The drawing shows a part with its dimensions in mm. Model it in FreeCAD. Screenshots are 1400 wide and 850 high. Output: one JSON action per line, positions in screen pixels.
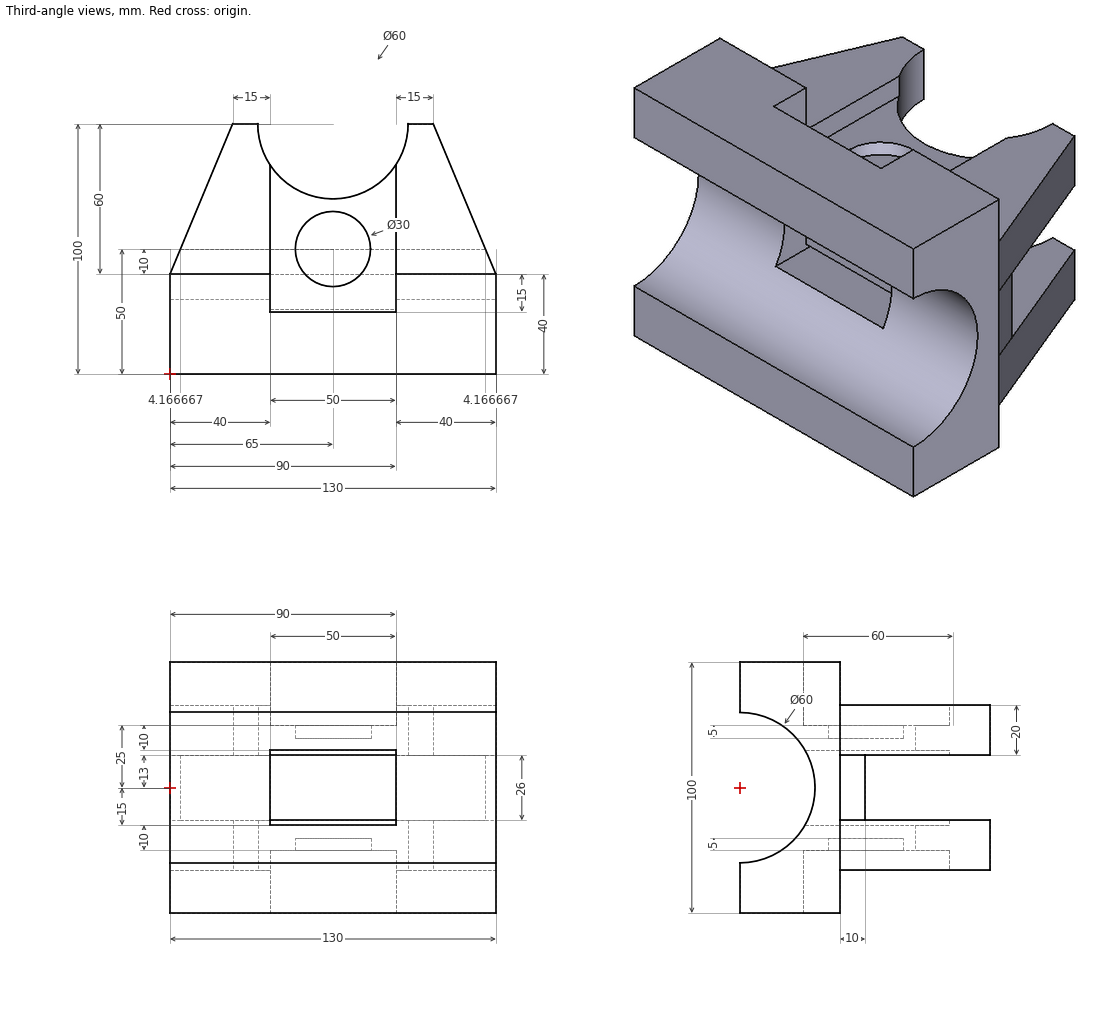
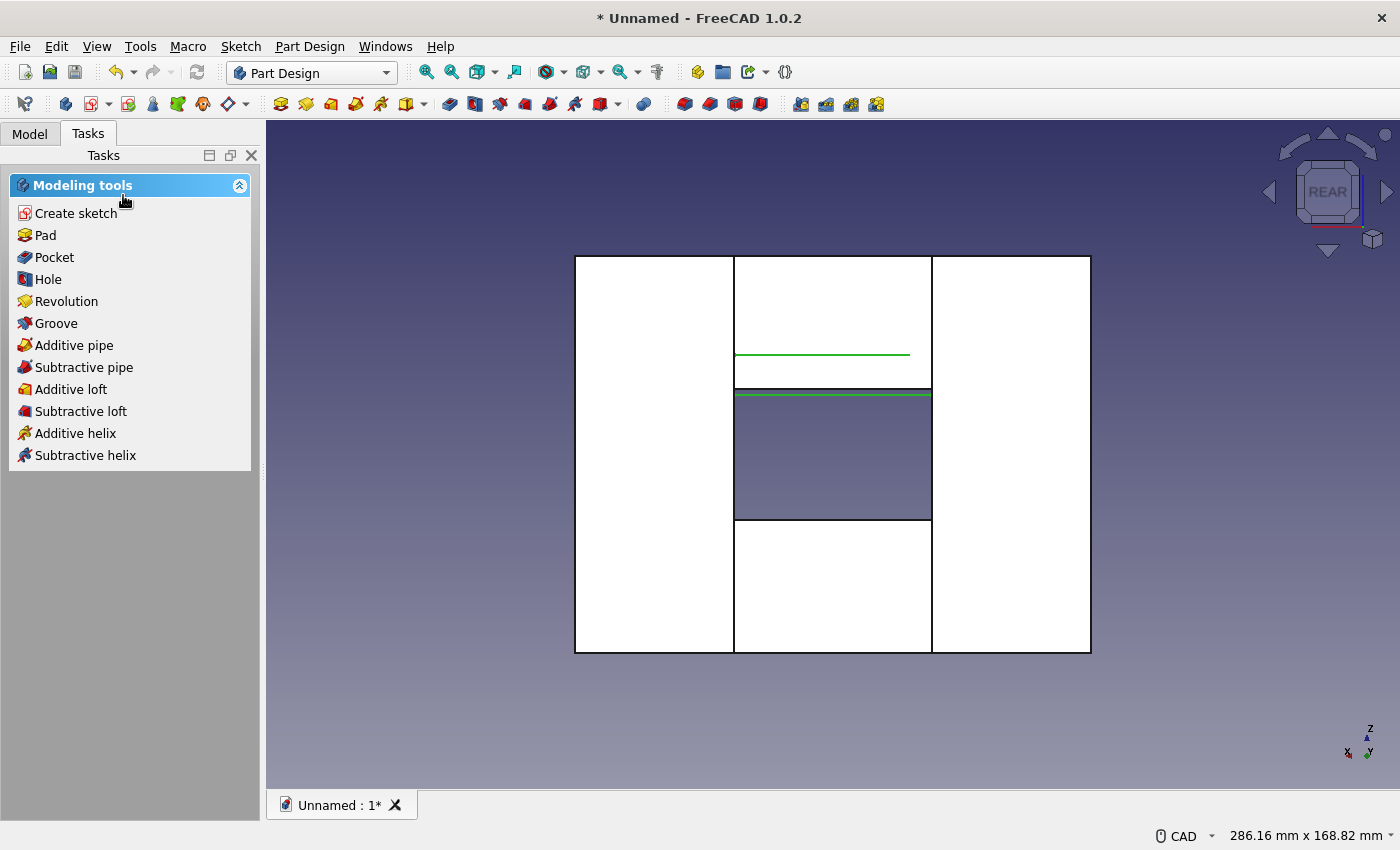
{"action": "left_click", "coordinate": [281, 104]}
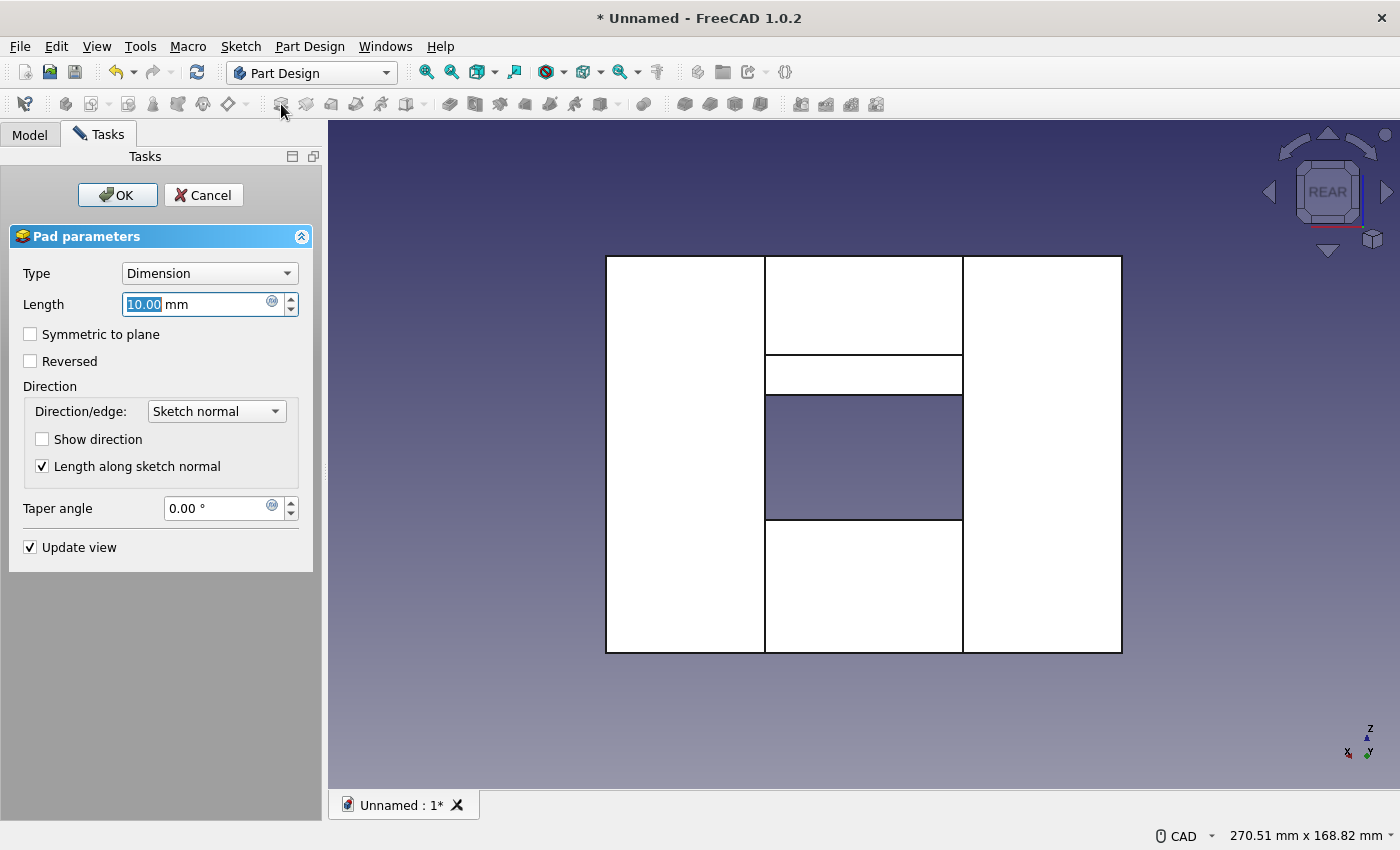
{"action": "type", "text": "60"}
{"action": "key", "text": "Tab"}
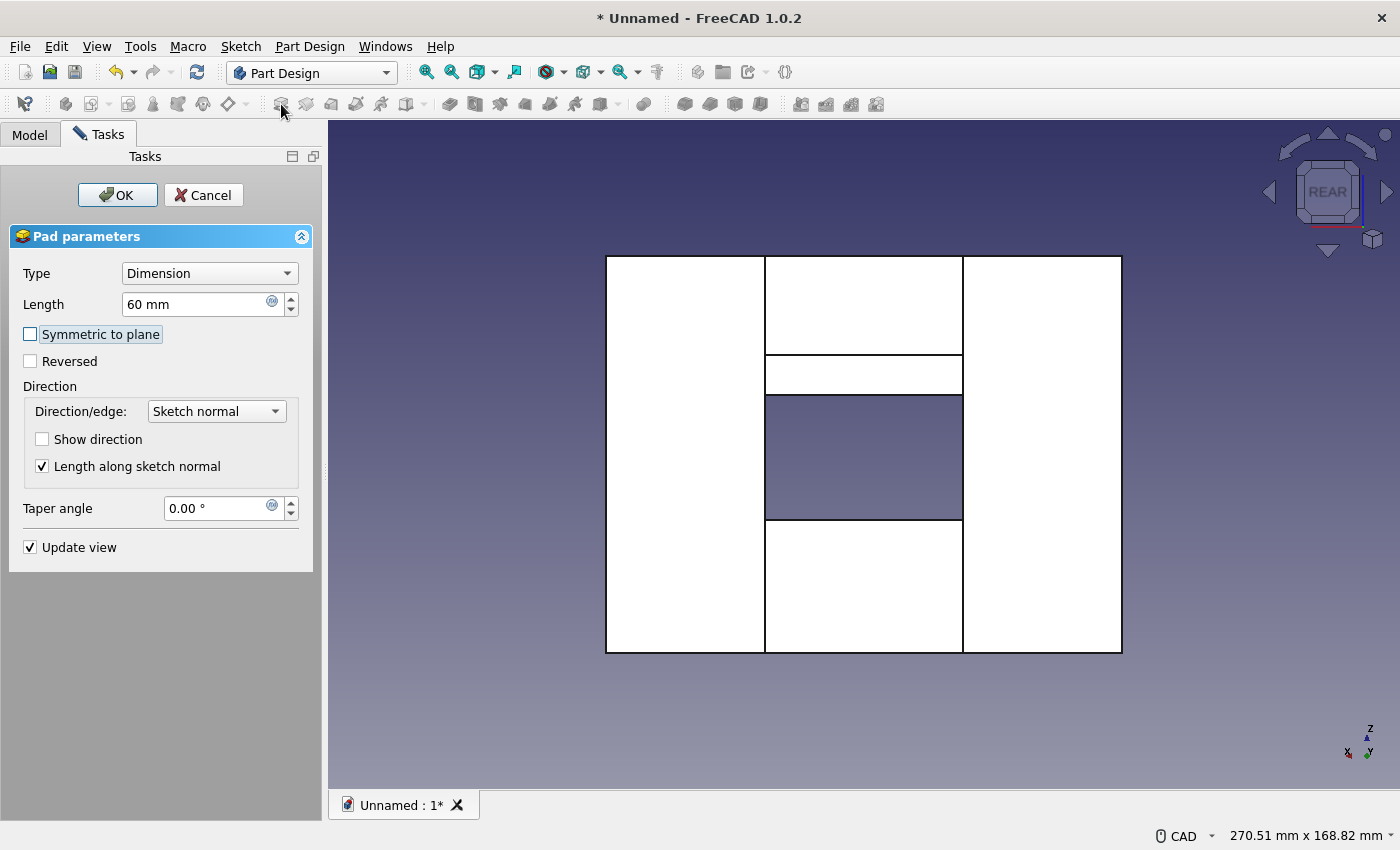
{"action": "left_click", "coordinate": [118, 195]}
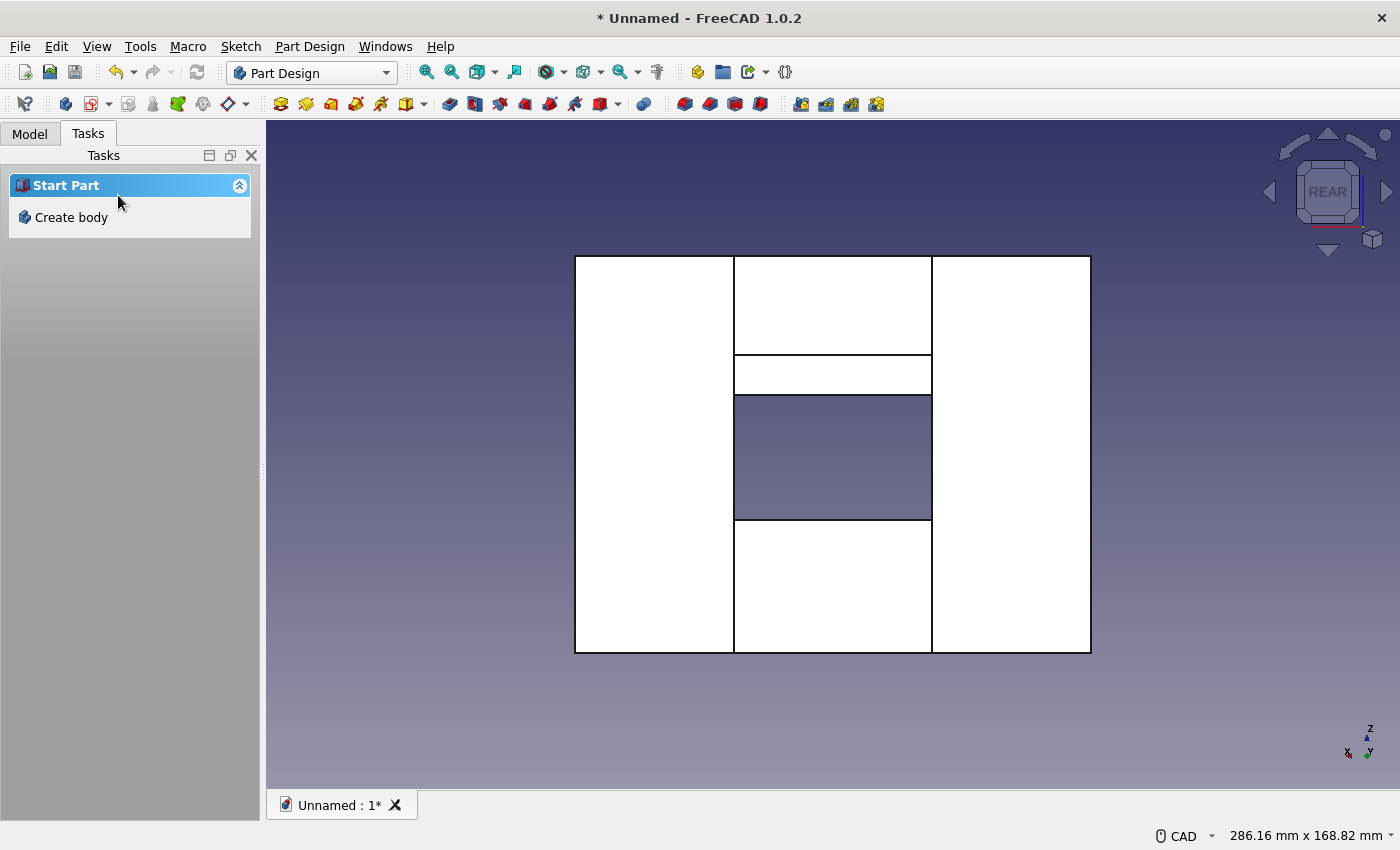
{"action": "left_click", "coordinate": [805, 585]}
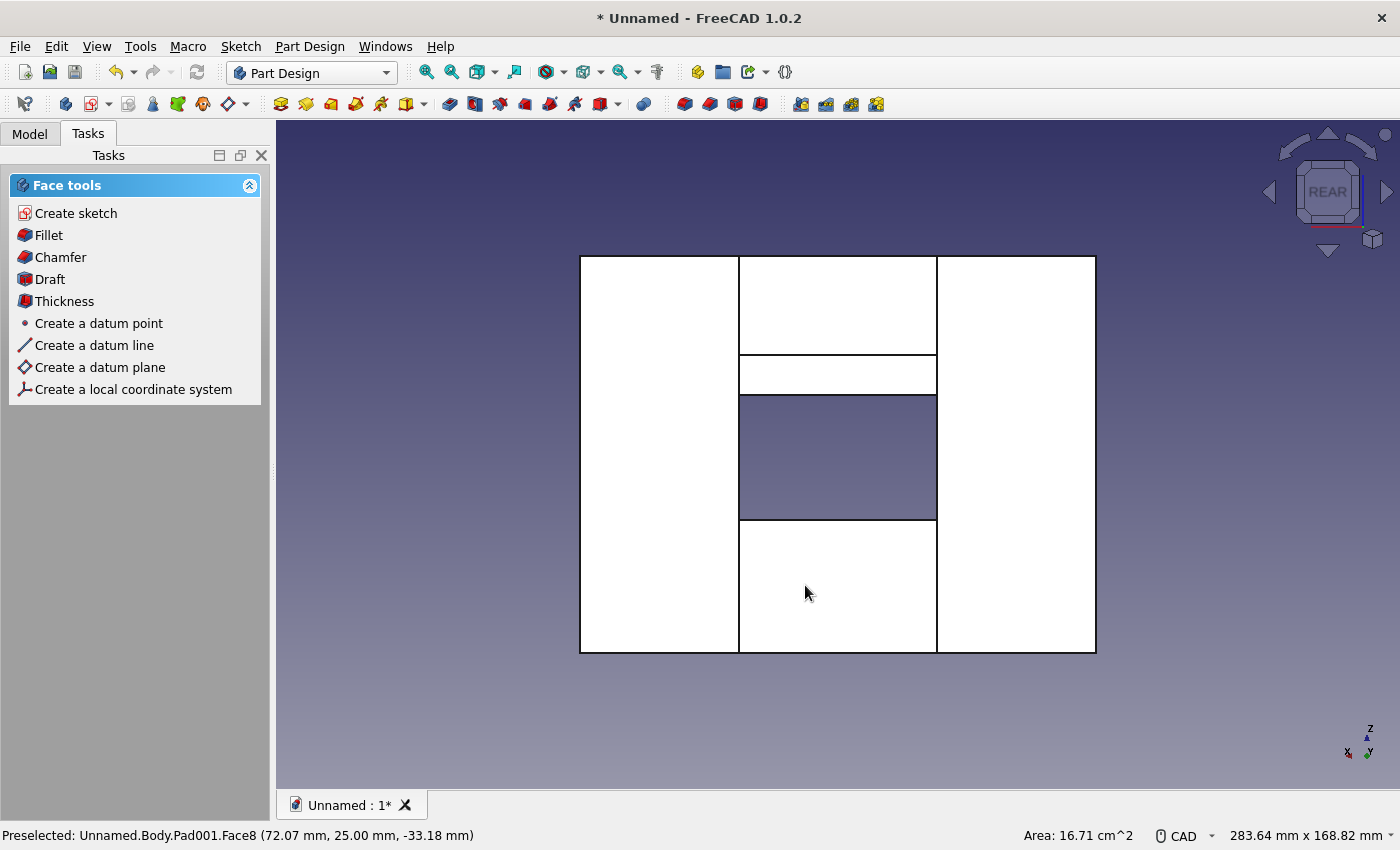
{"action": "left_click", "coordinate": [90, 104]}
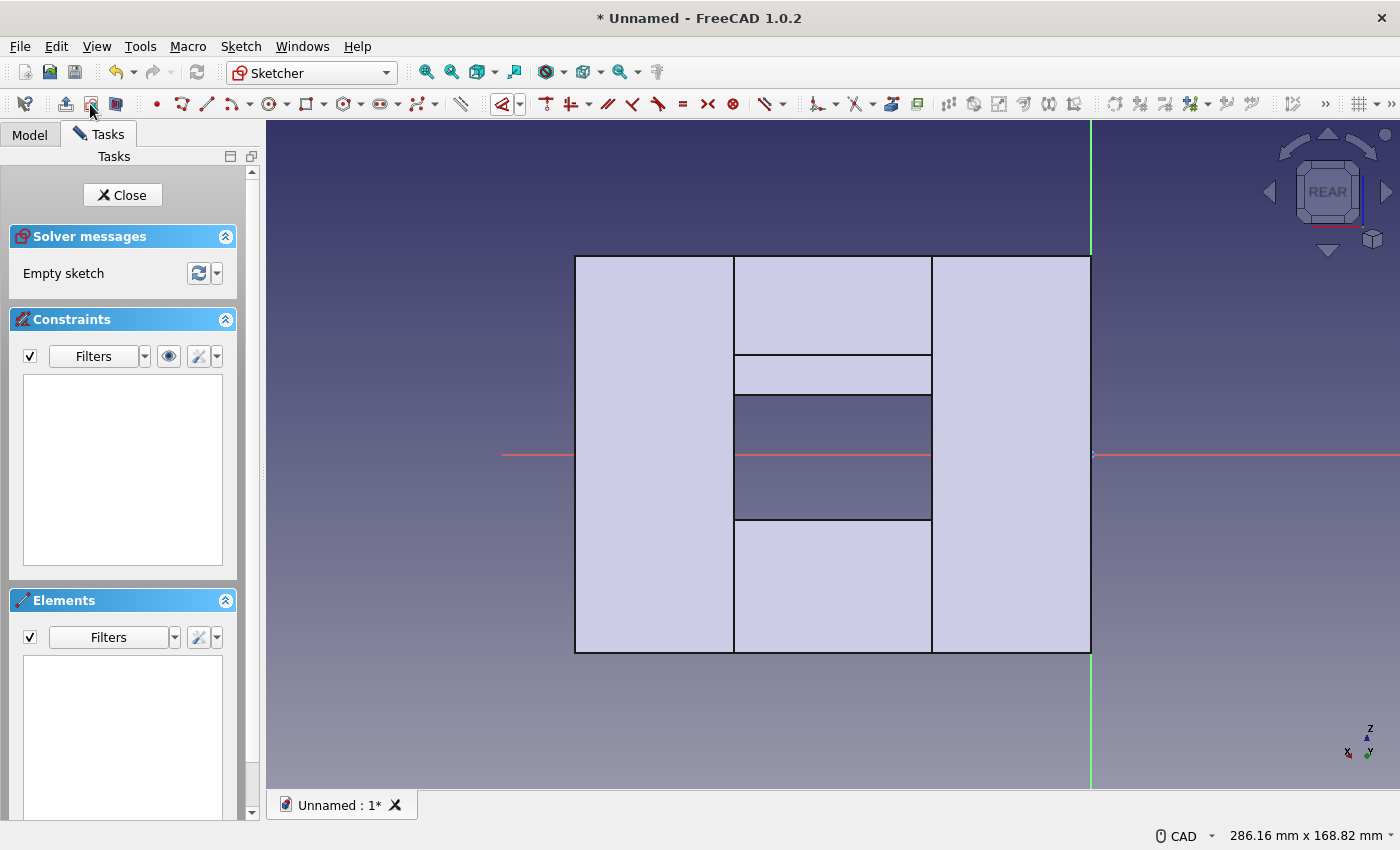
{"action": "scroll", "coordinate": [1092, 564], "scroll_direction": "up", "scroll_amount": 3}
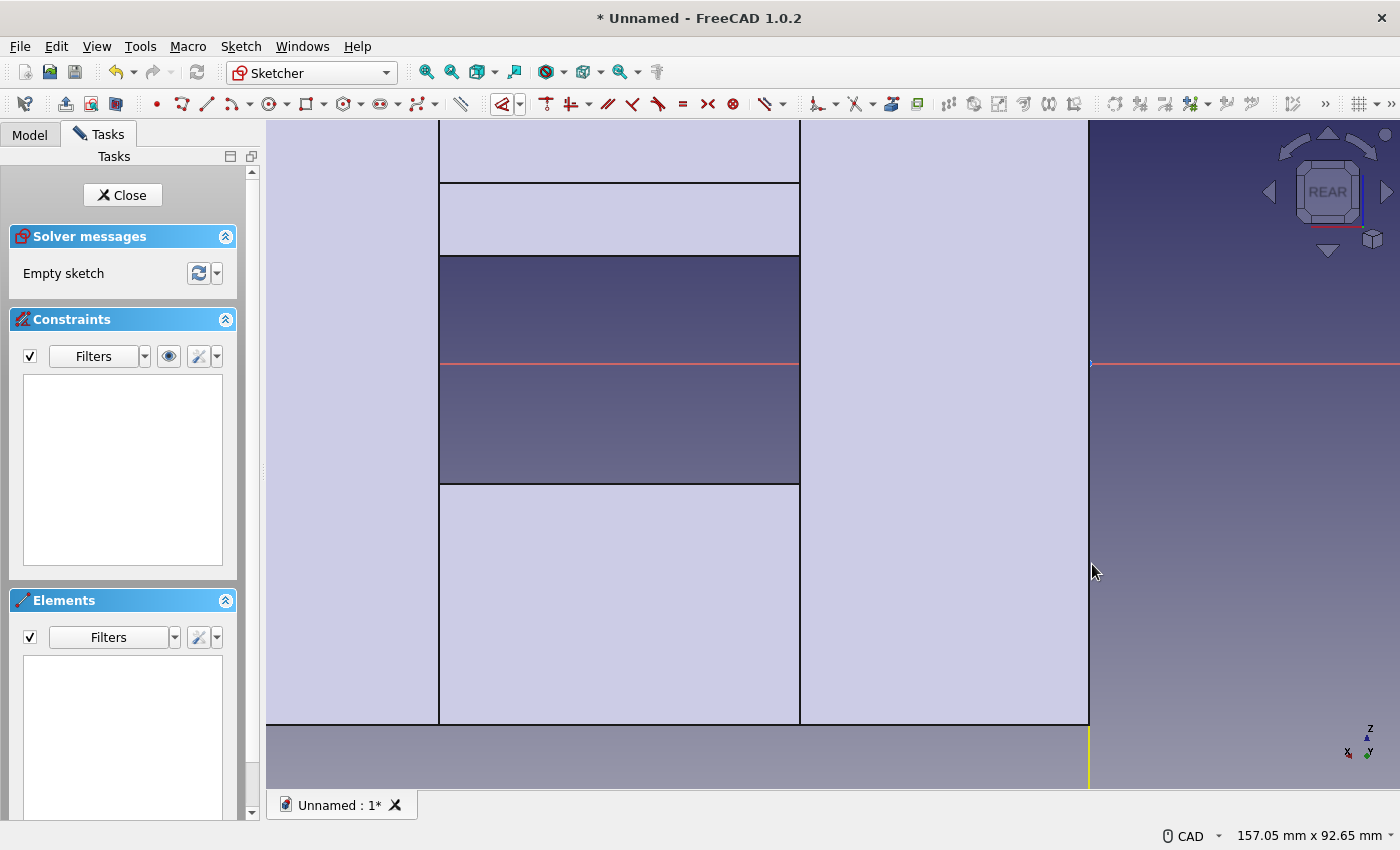
{"action": "left_click", "coordinate": [306, 104]}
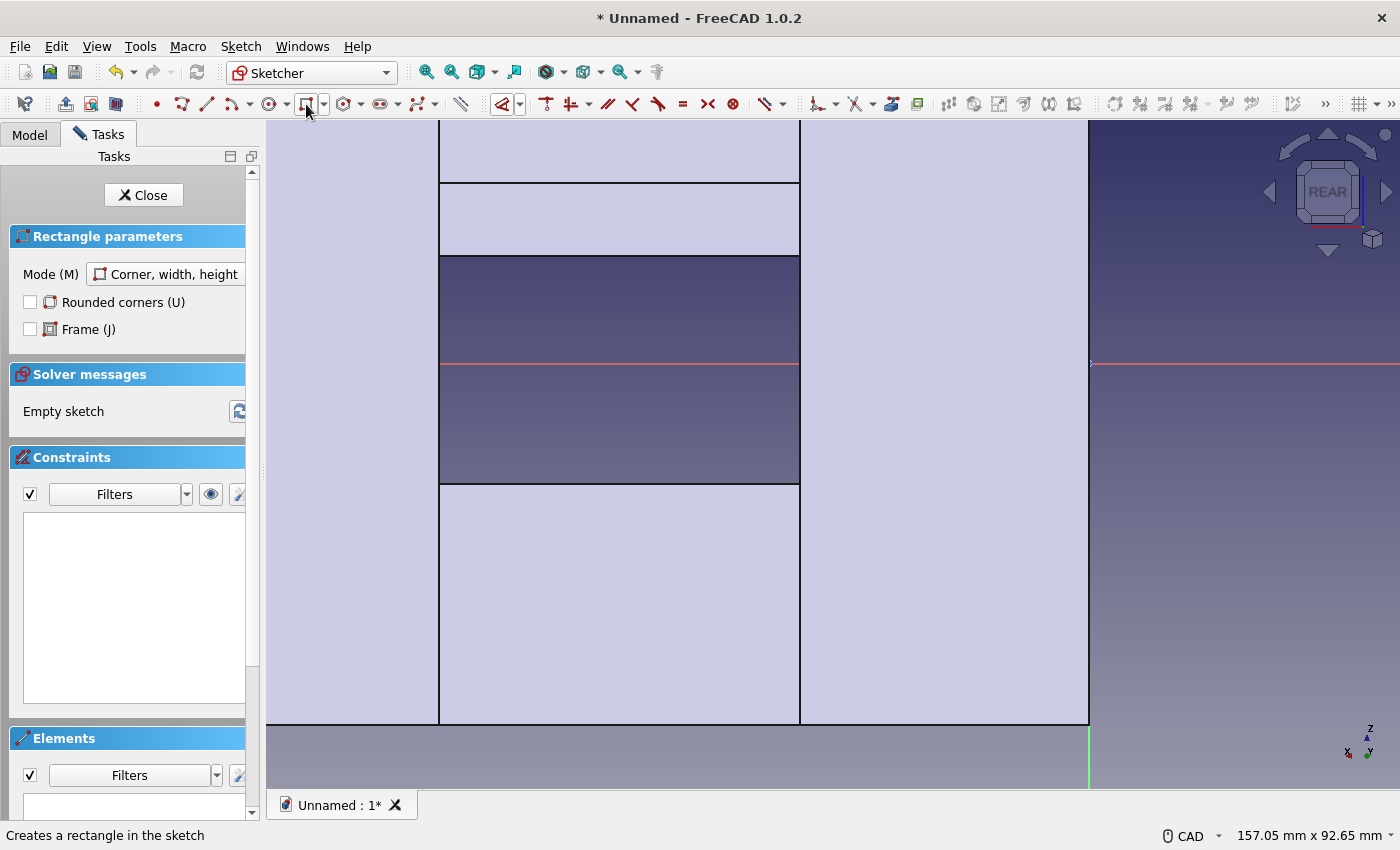
{"action": "left_click", "coordinate": [439, 472]}
{"action": "mouse_move", "coordinate": [800, 544]}